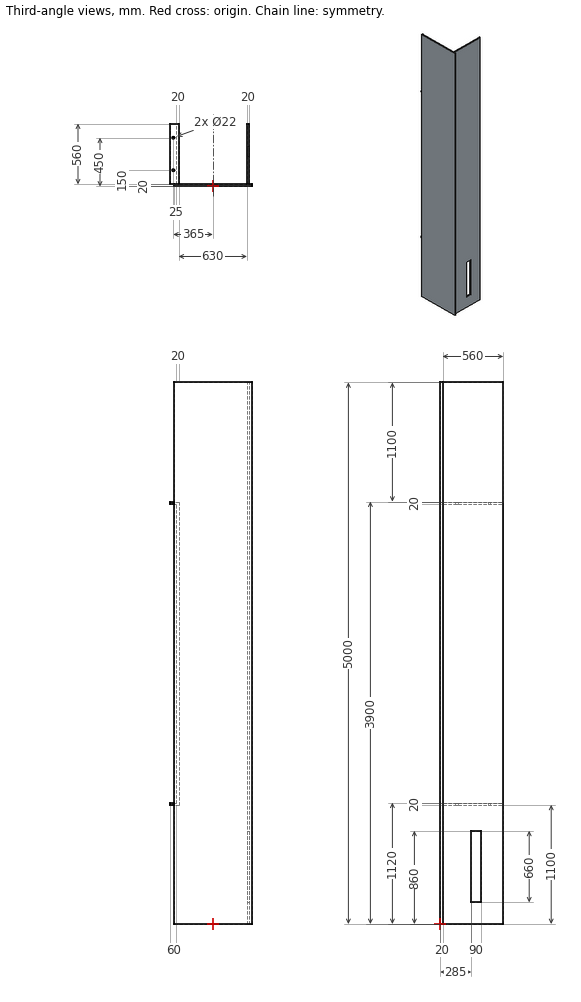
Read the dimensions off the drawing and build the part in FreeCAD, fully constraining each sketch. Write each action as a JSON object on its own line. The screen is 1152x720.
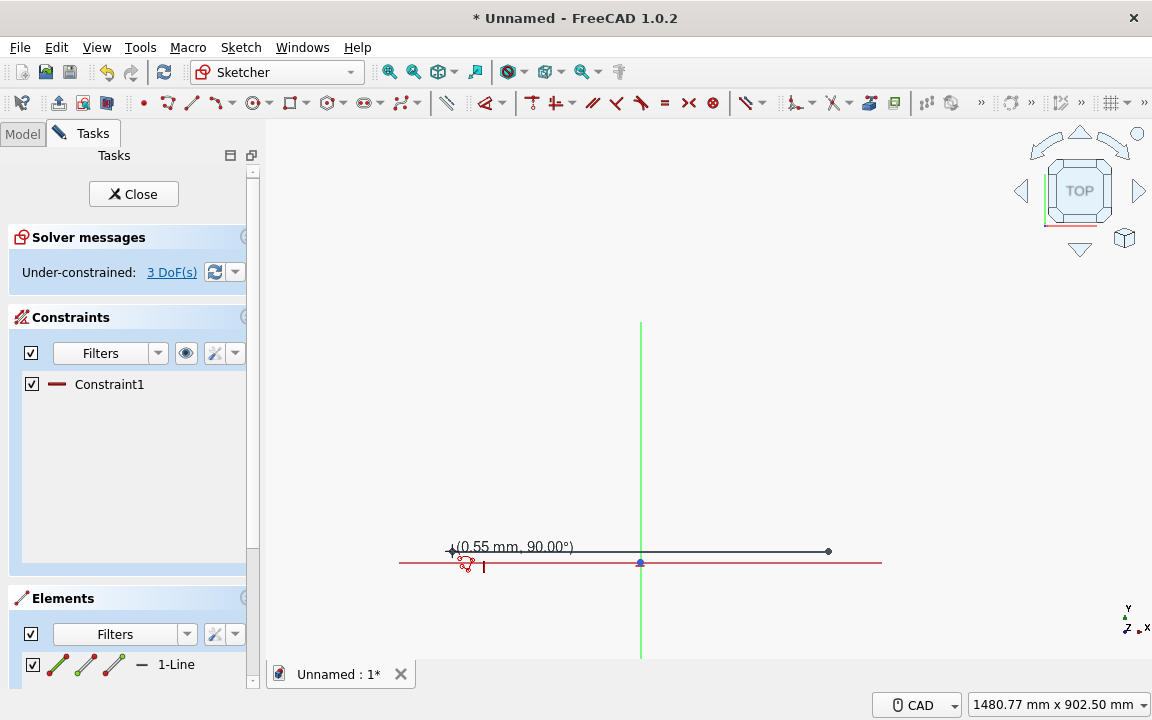
{"action": "left_click", "coordinate": [452, 216]}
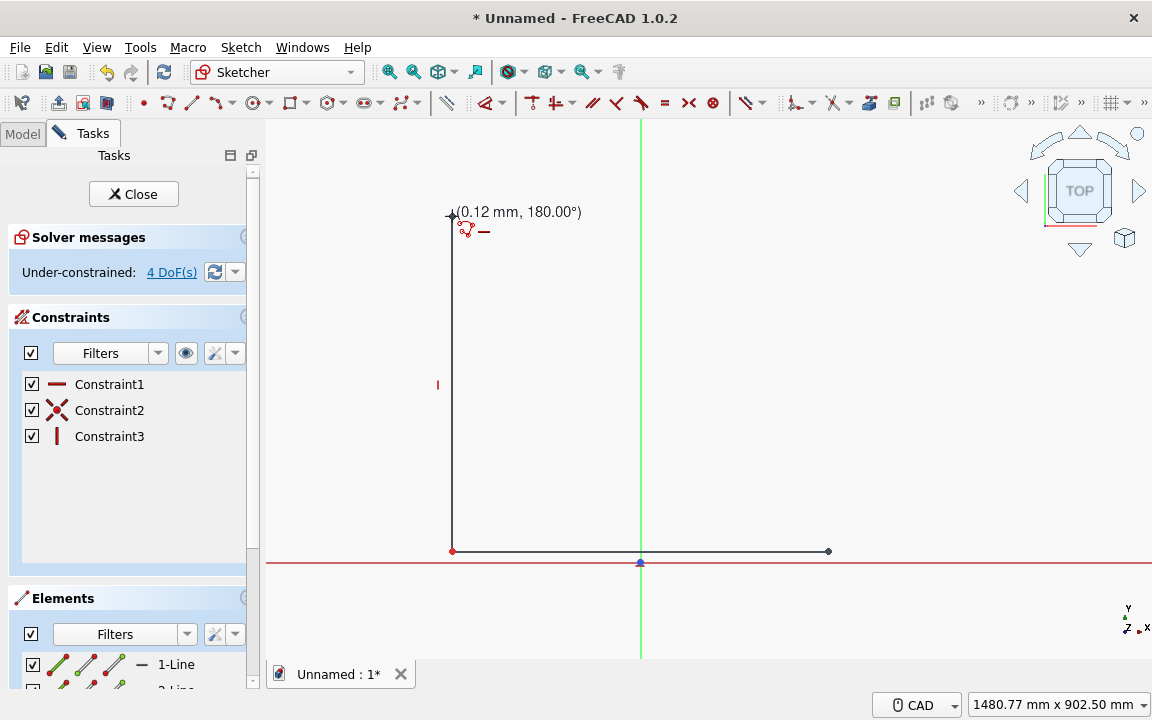
{"action": "scroll", "coordinate": [440, 216], "scroll_direction": "up", "scroll_amount": 2}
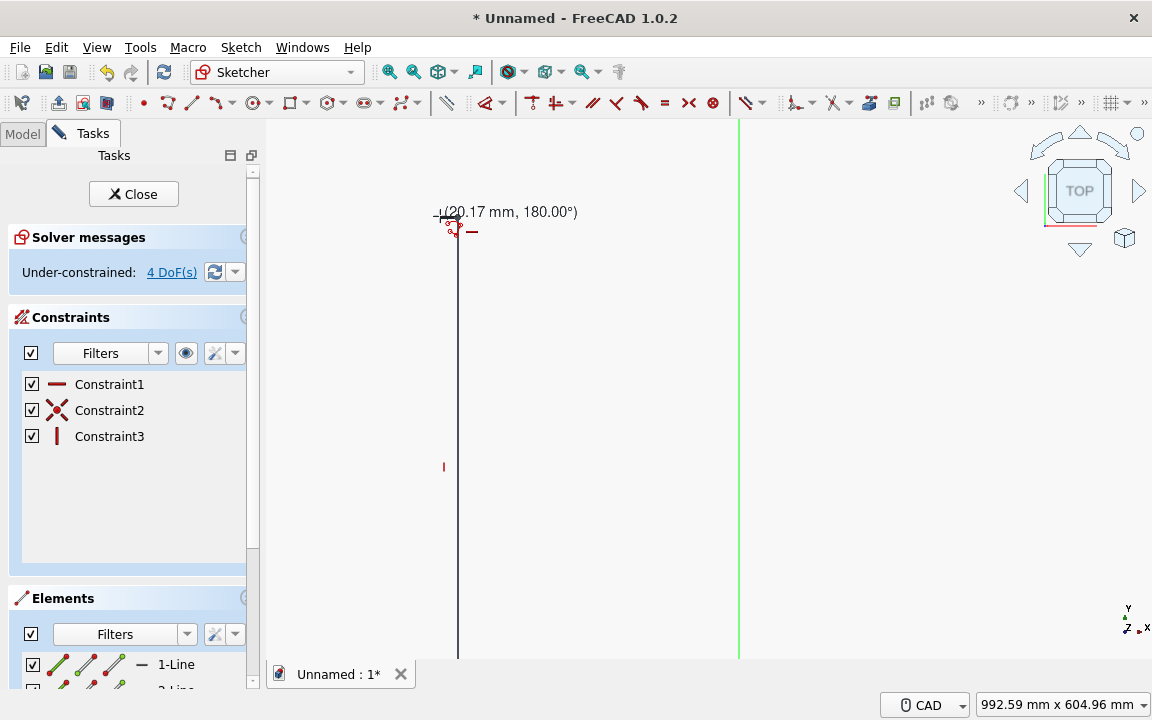
{"action": "left_click", "coordinate": [440, 216]}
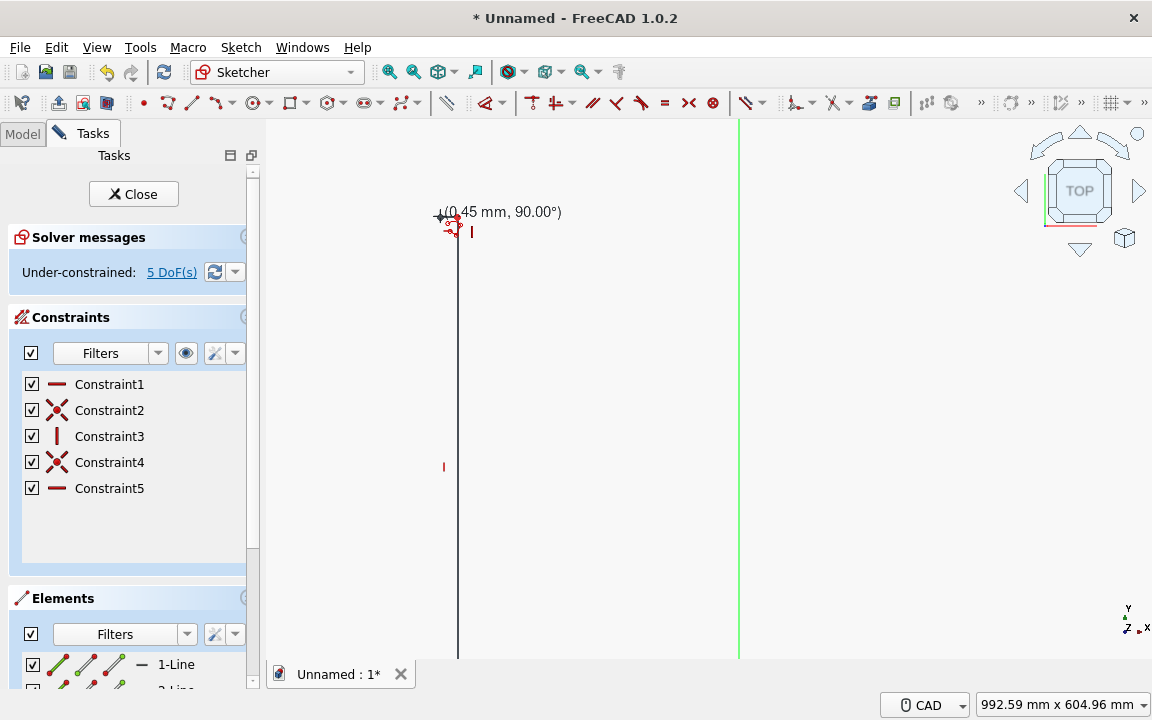
{"action": "scroll", "coordinate": [440, 215], "scroll_direction": "down", "scroll_amount": 2}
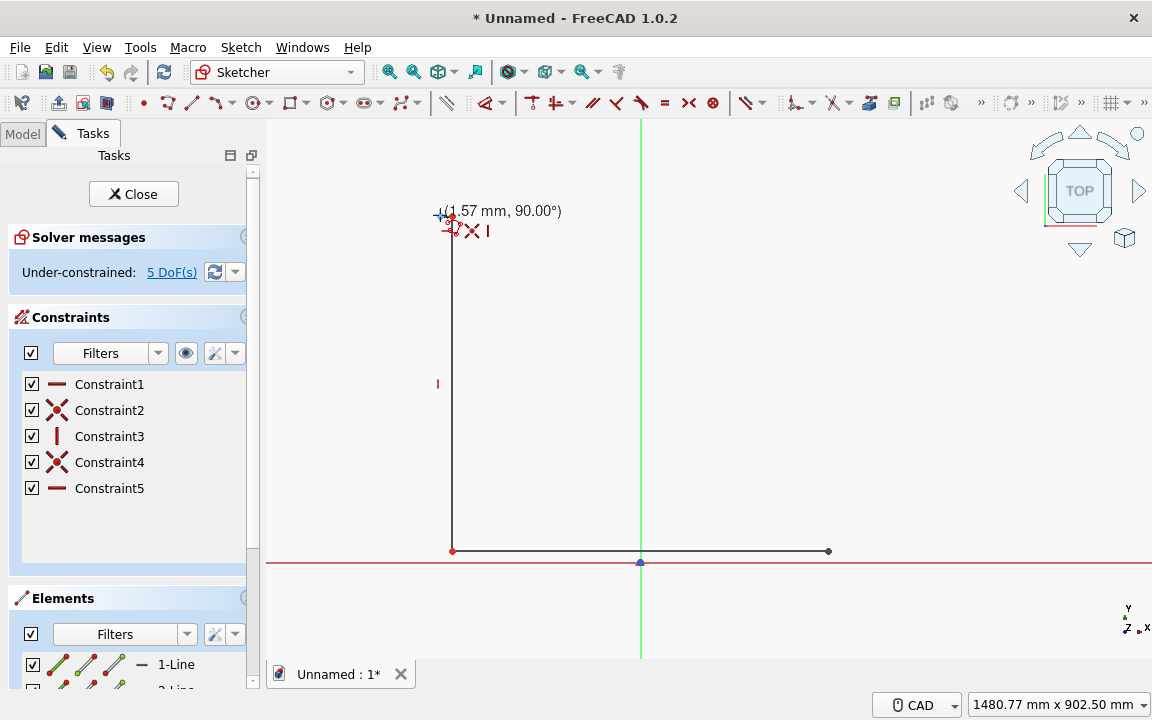
{"action": "scroll", "coordinate": [440, 551], "scroll_direction": "up", "scroll_amount": 2}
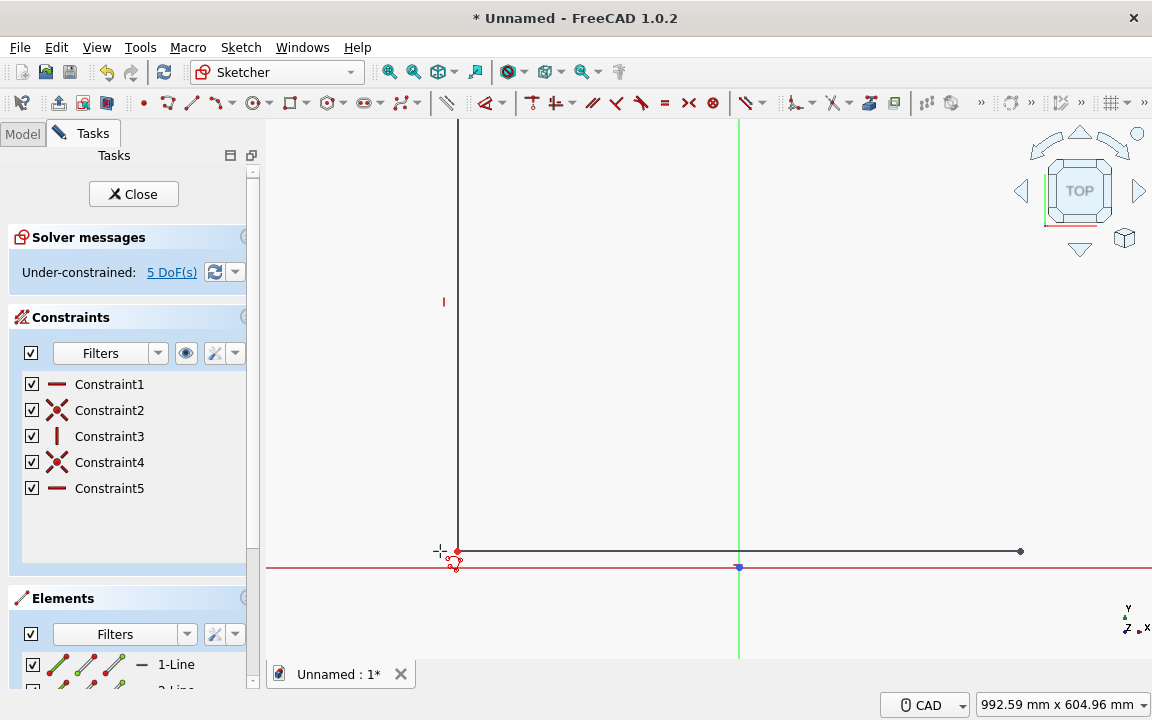
{"action": "left_click", "coordinate": [440, 550]}
{"action": "left_click", "coordinate": [418, 550]}
{"action": "left_click", "coordinate": [418, 568]}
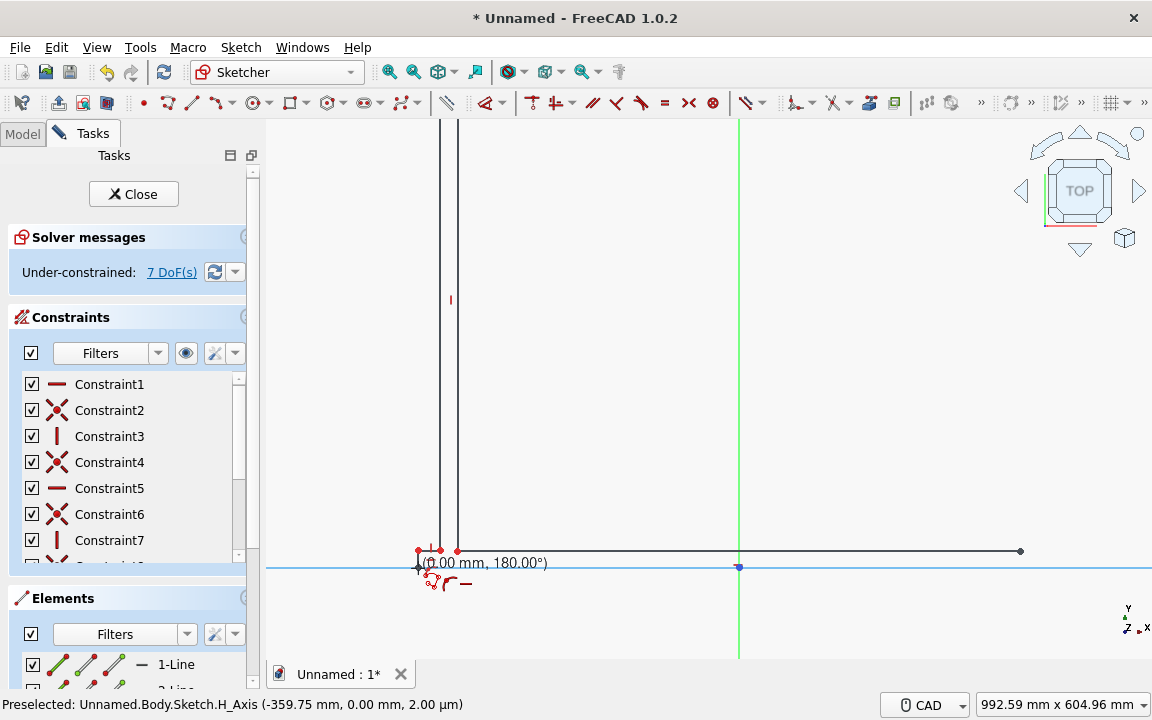
{"action": "scroll", "coordinate": [440, 552], "scroll_direction": "down", "scroll_amount": 2}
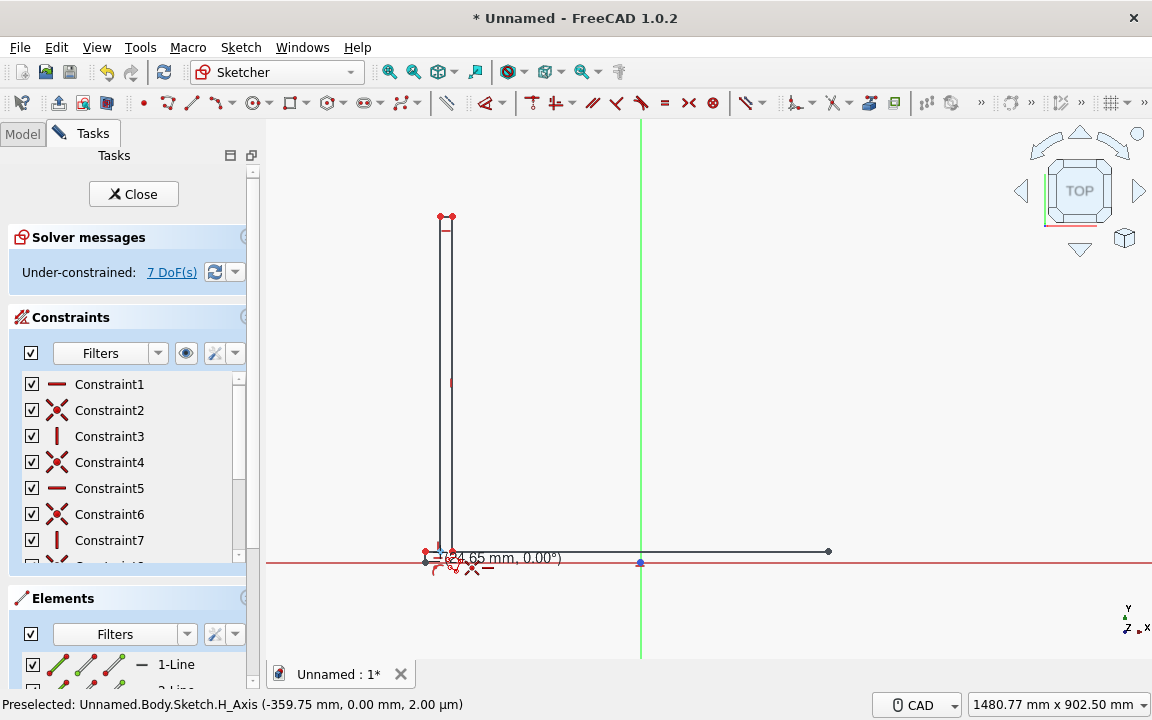
{"action": "left_click", "coordinate": [856, 554]}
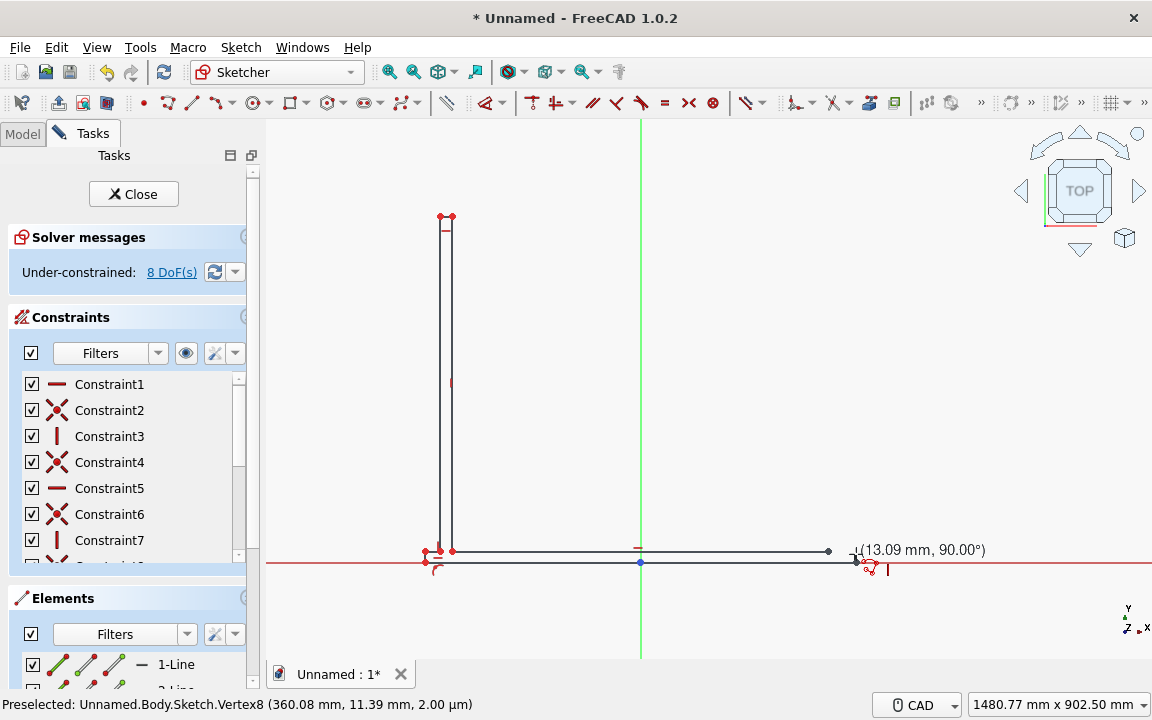
{"action": "scroll", "coordinate": [856, 551], "scroll_direction": "up", "scroll_amount": 2}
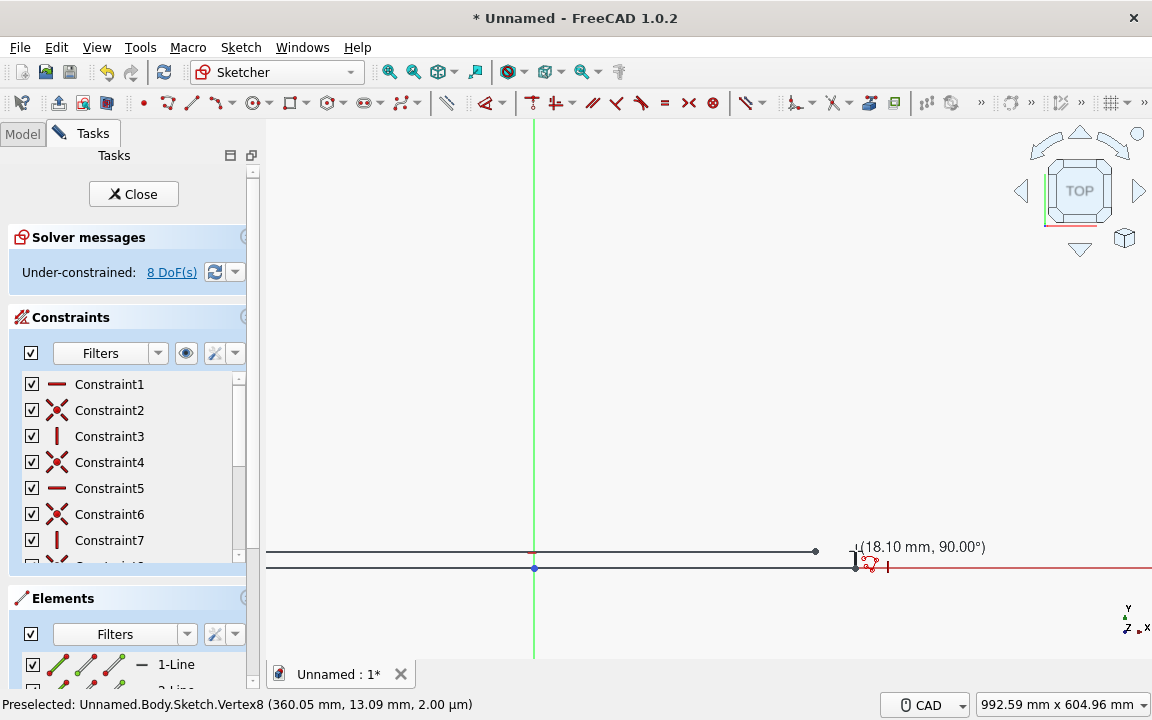
{"action": "left_click", "coordinate": [856, 550]}
{"action": "left_click", "coordinate": [833, 550]}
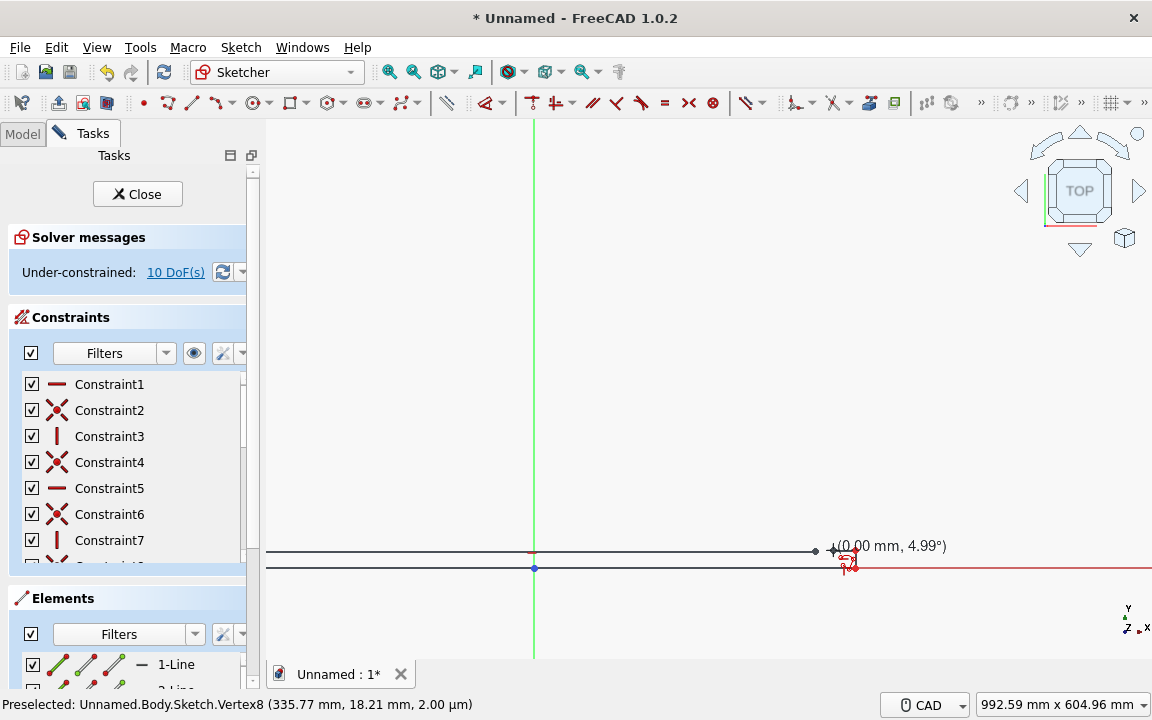
{"action": "scroll", "coordinate": [856, 551], "scroll_direction": "down", "scroll_amount": 2}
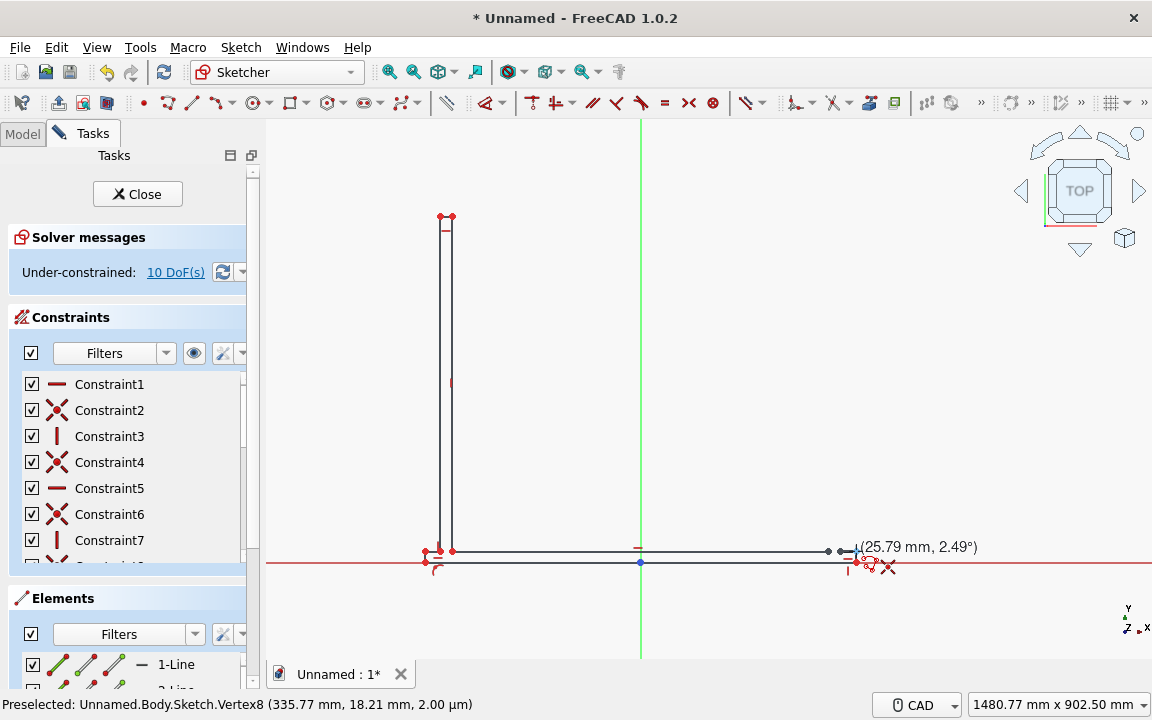
{"action": "left_click", "coordinate": [841, 216]}